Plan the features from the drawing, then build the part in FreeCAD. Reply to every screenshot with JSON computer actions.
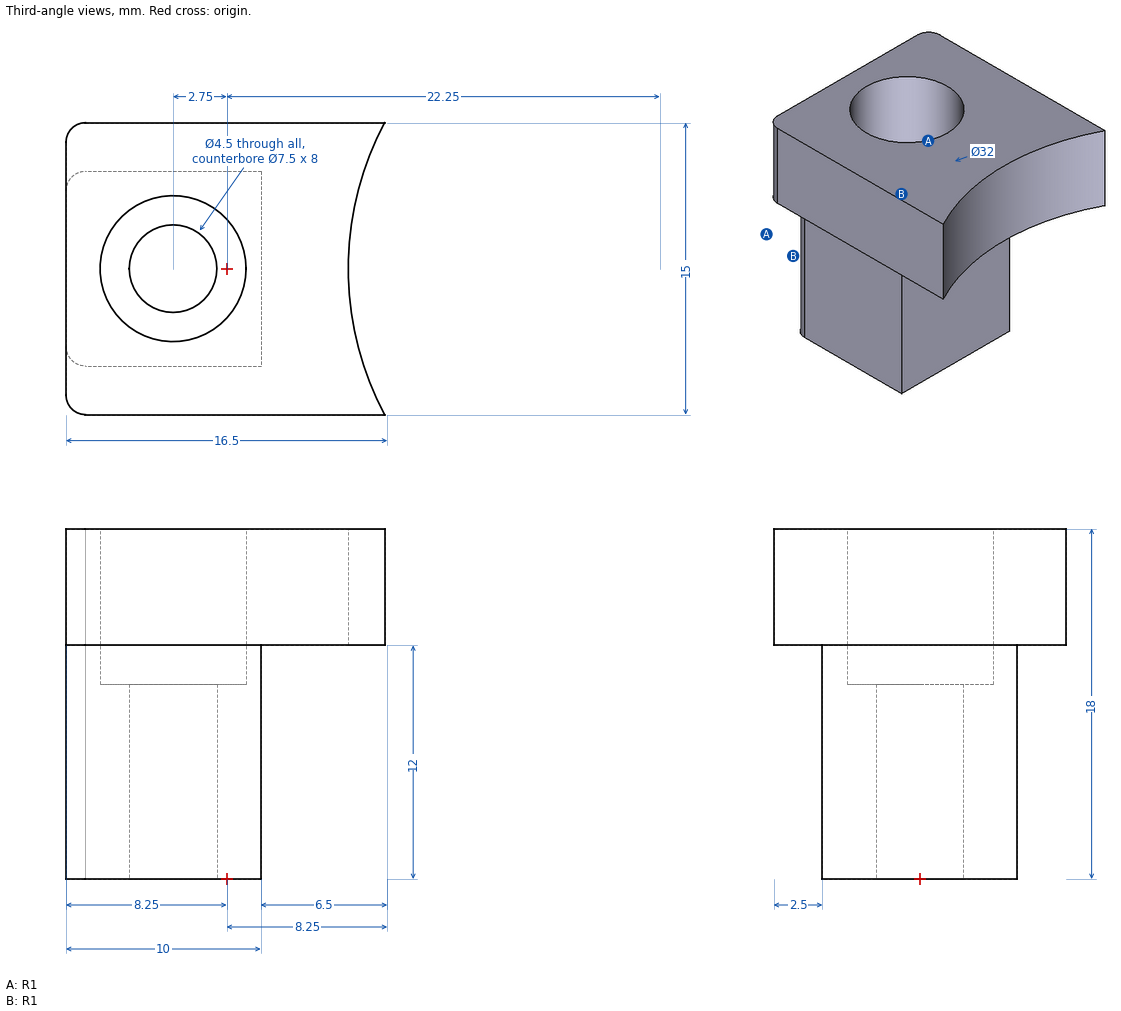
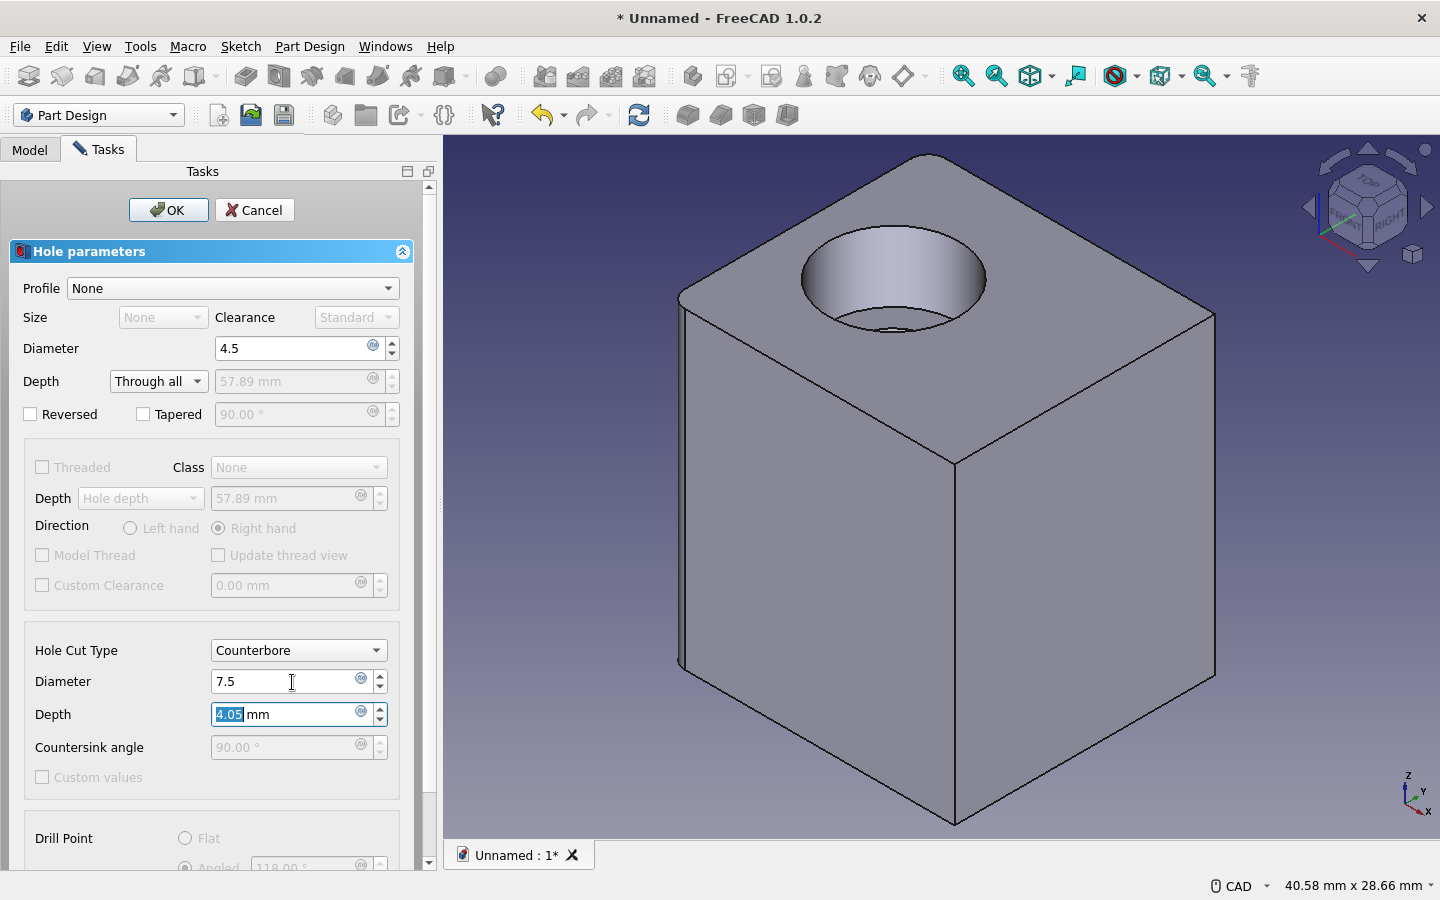
{"action": "type", "text": "8"}
{"action": "key", "text": "Tab"}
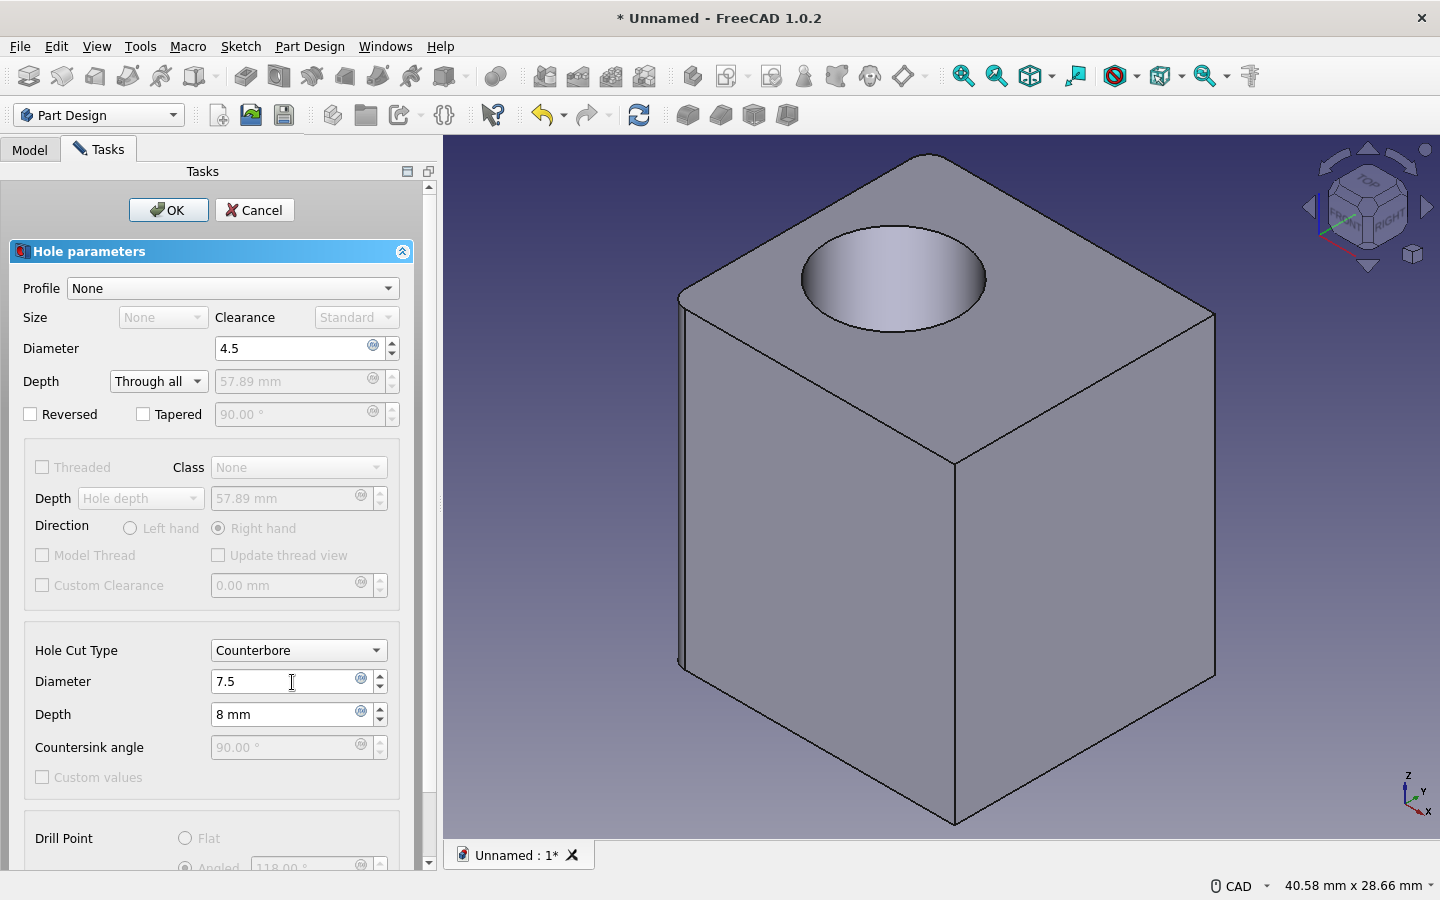
{"action": "left_click", "coordinate": [169, 210]}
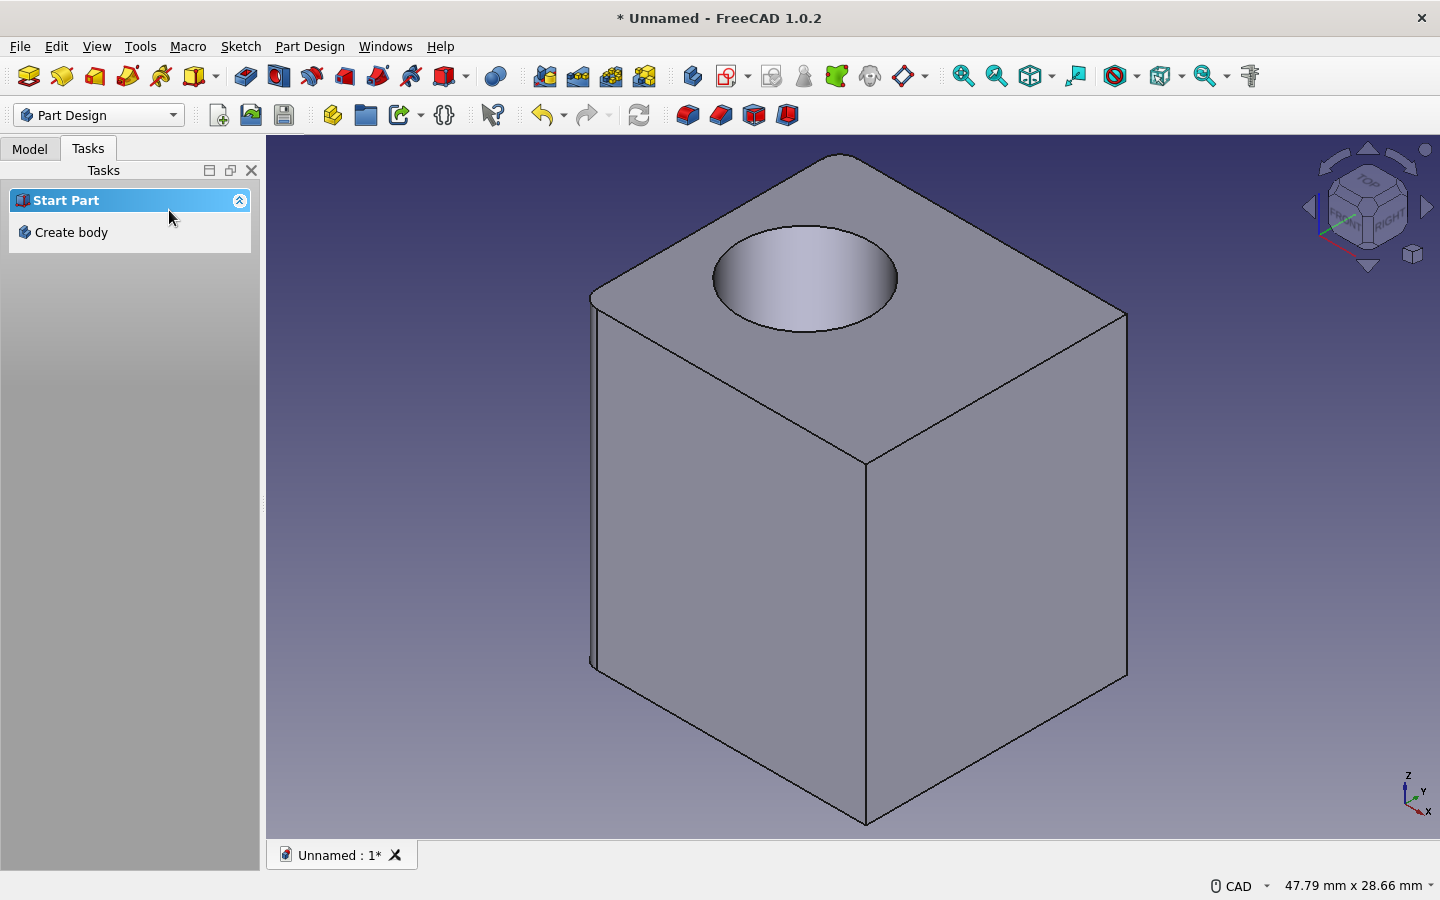
{"action": "left_click", "coordinate": [972, 331]}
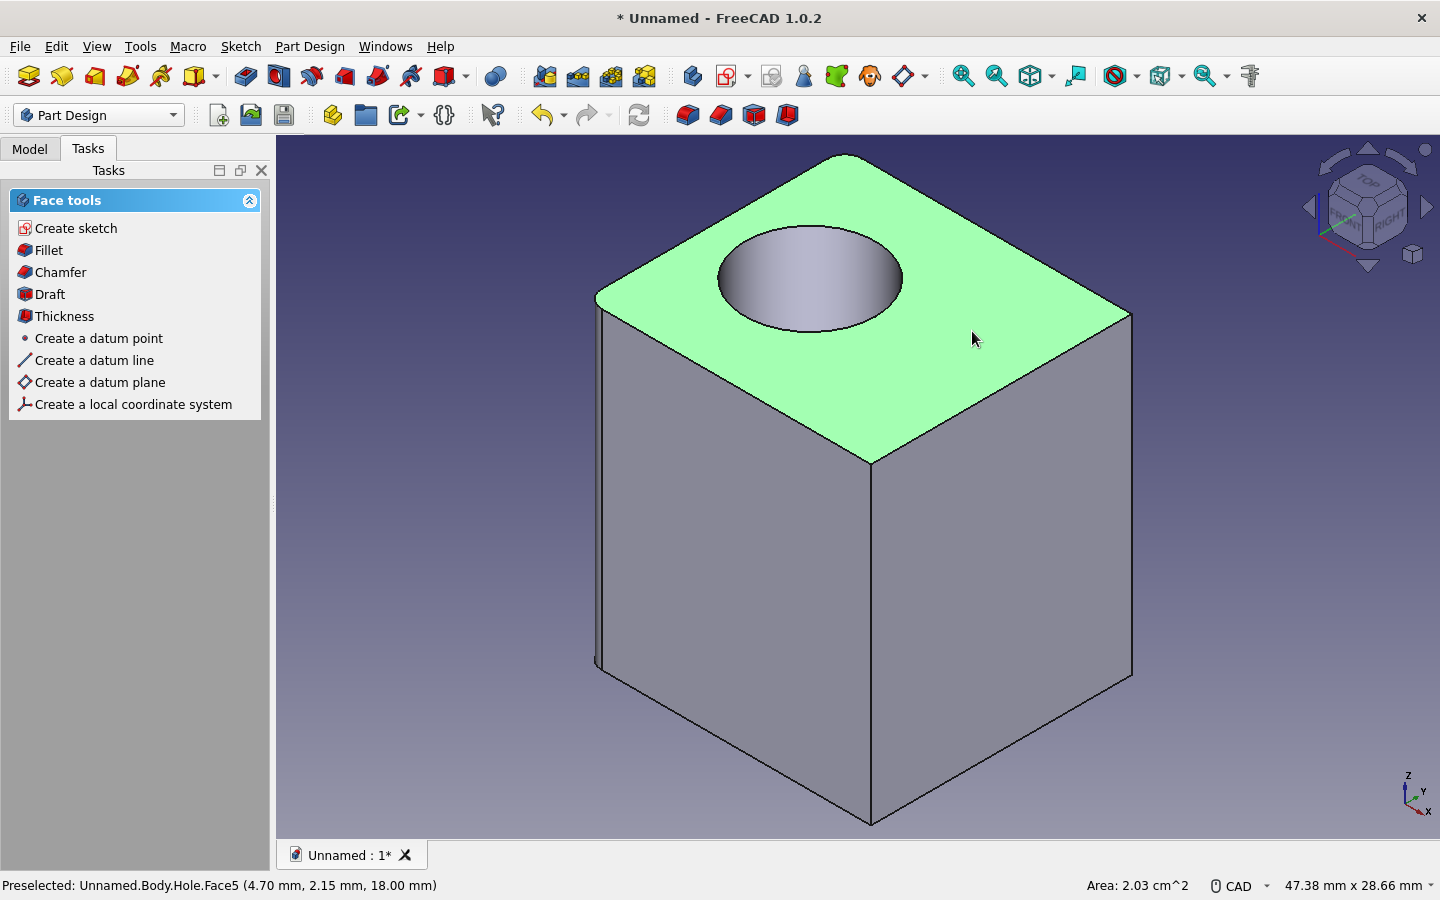
{"action": "left_click", "coordinate": [726, 76]}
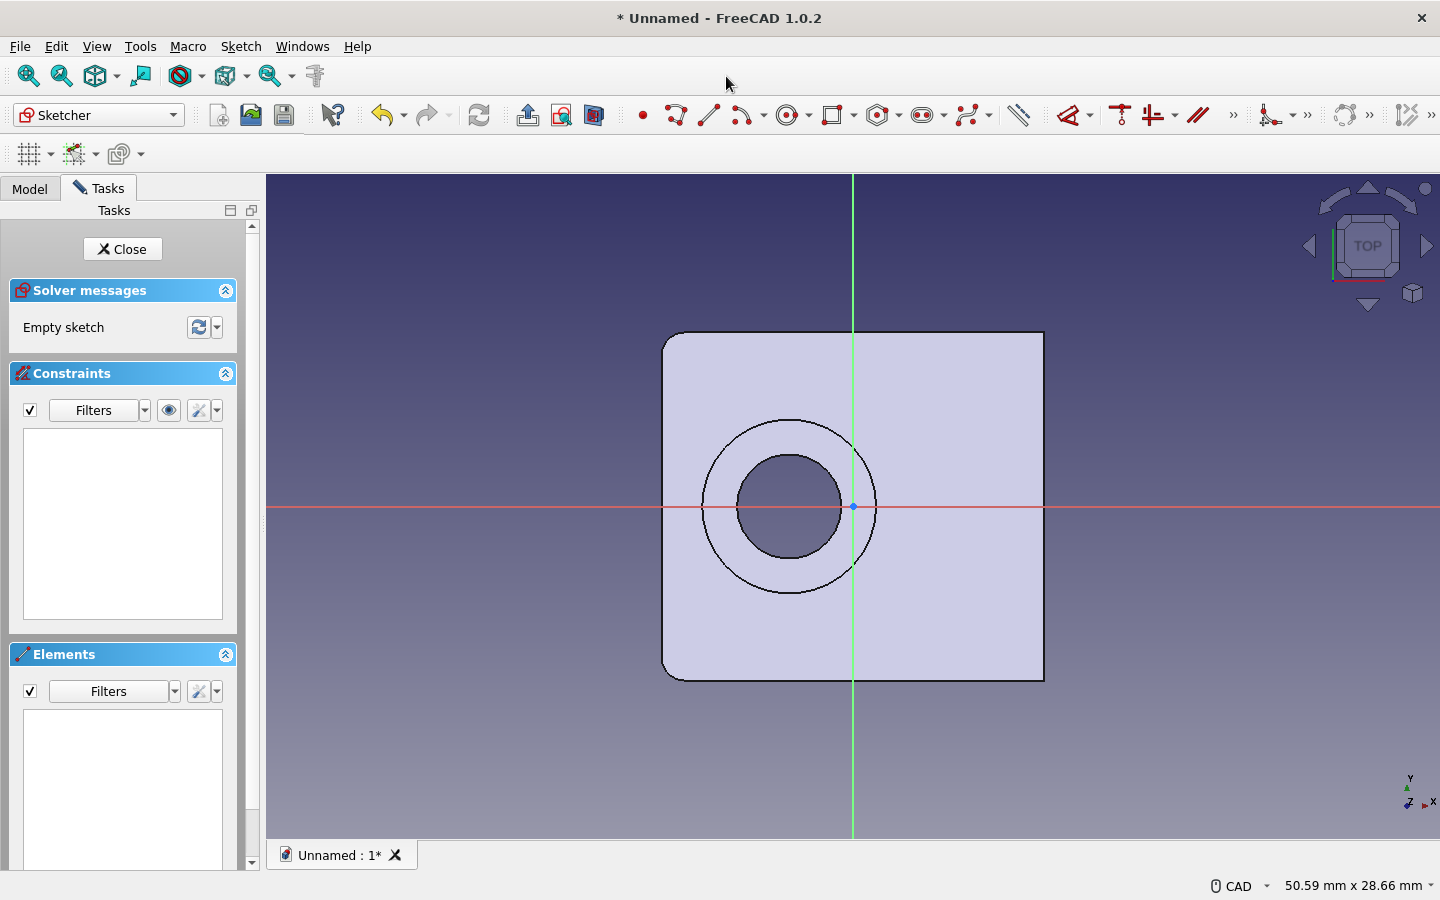
{"action": "scroll", "coordinate": [294, 507], "scroll_direction": "down", "scroll_amount": 3}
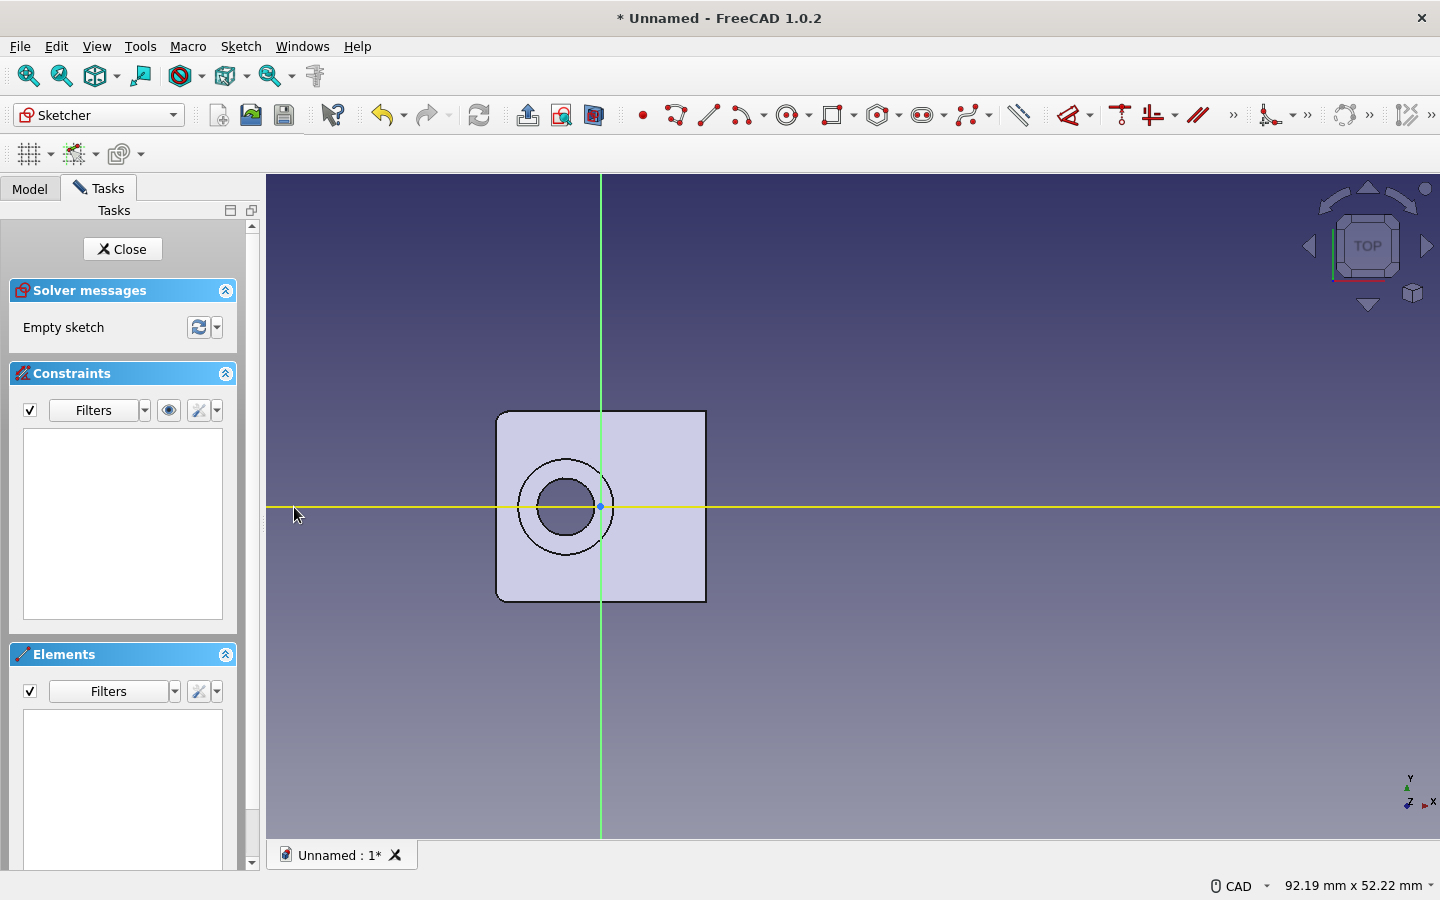
{"action": "left_click", "coordinate": [786, 116]}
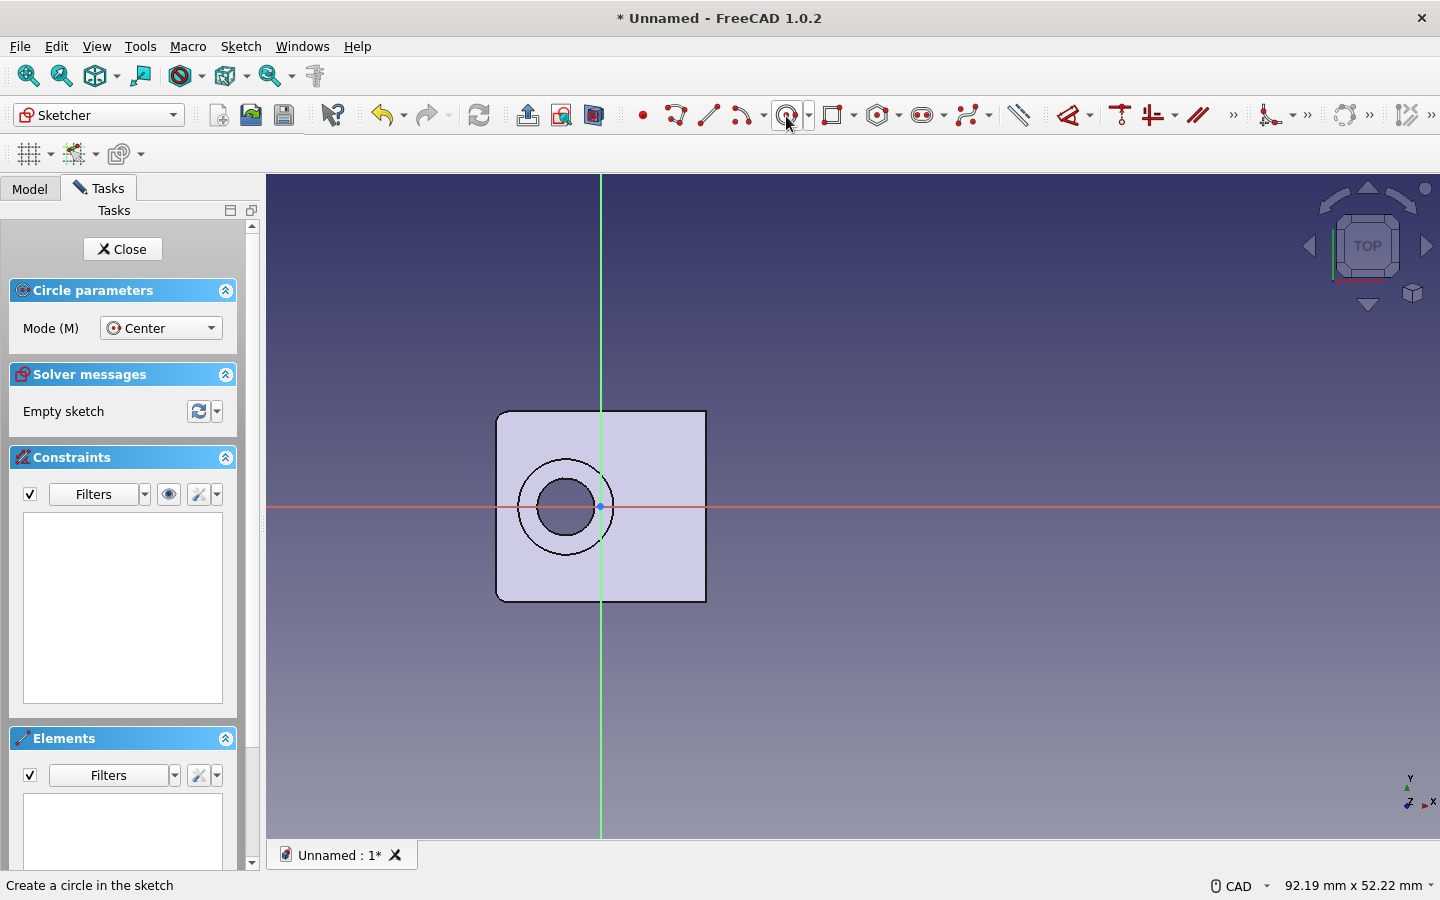
{"action": "left_click", "coordinate": [884, 507]}
{"action": "left_click", "coordinate": [1028, 363]}
{"action": "key", "text": "Escape"}